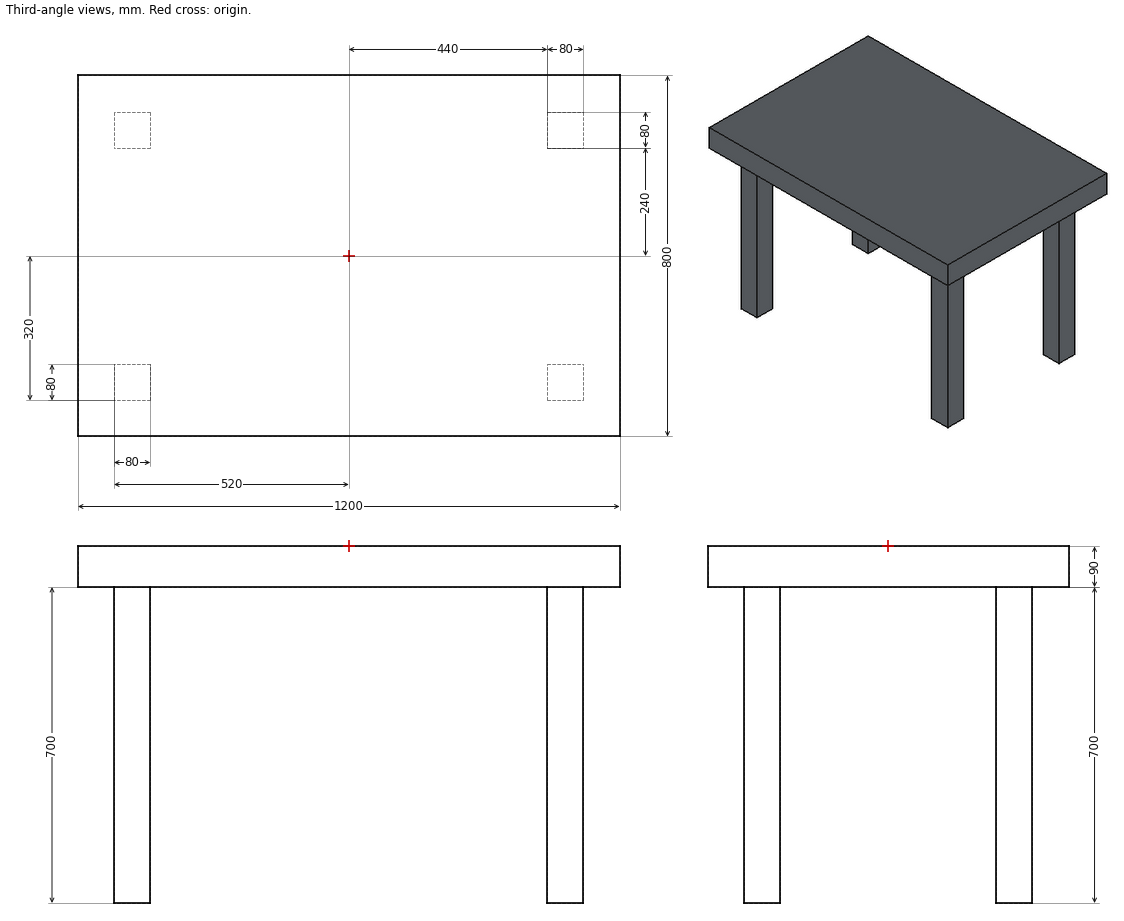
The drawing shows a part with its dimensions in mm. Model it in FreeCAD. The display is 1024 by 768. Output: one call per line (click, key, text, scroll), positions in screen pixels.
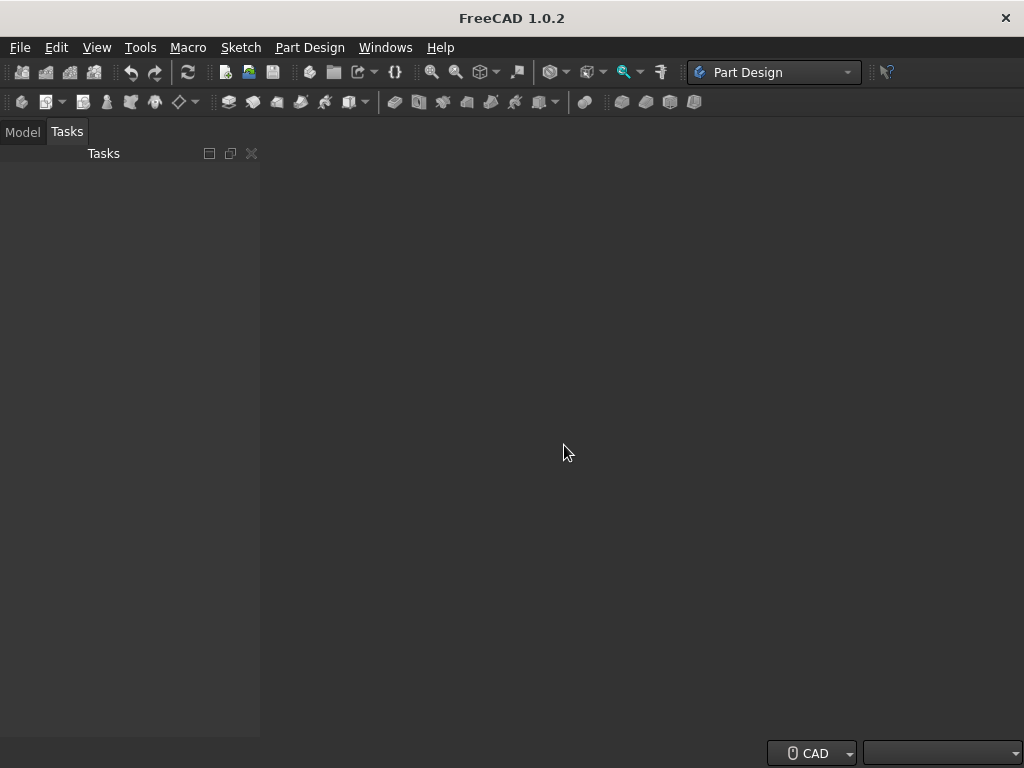
key(ctrl+n)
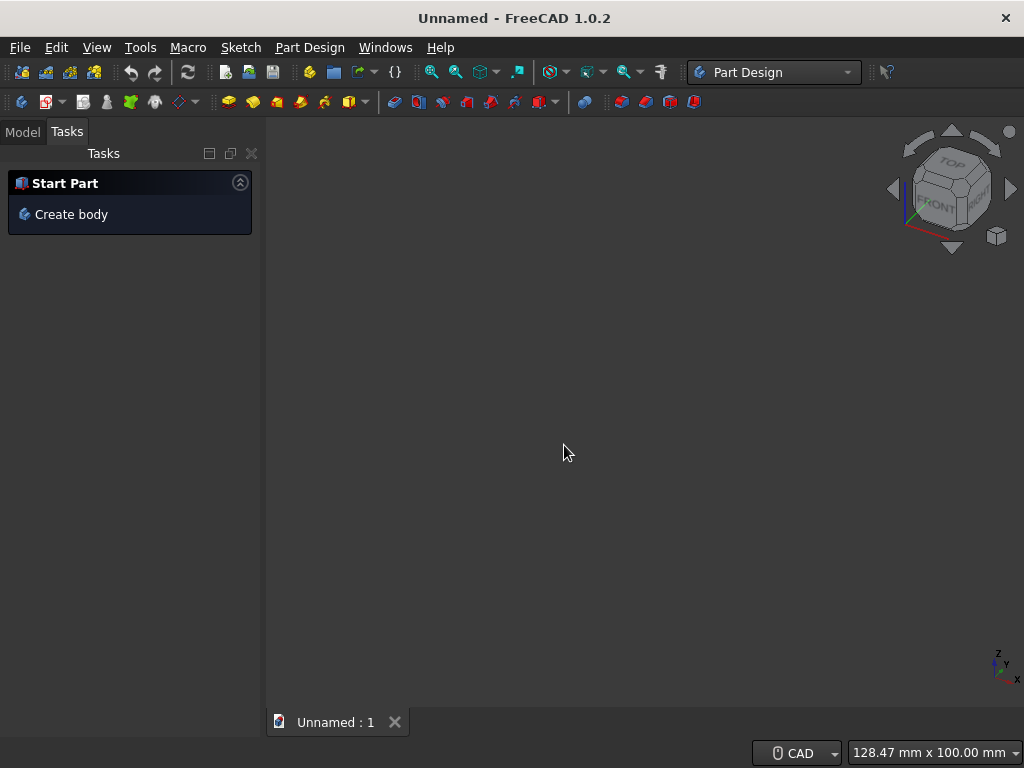
click(46, 102)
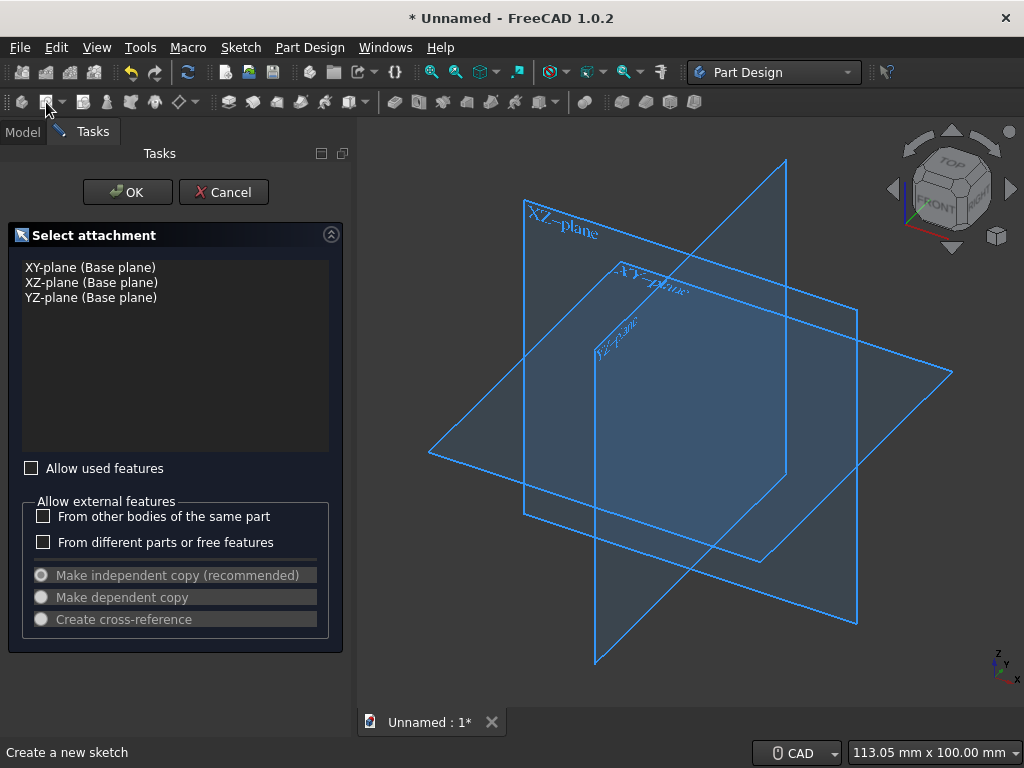
click(82, 268)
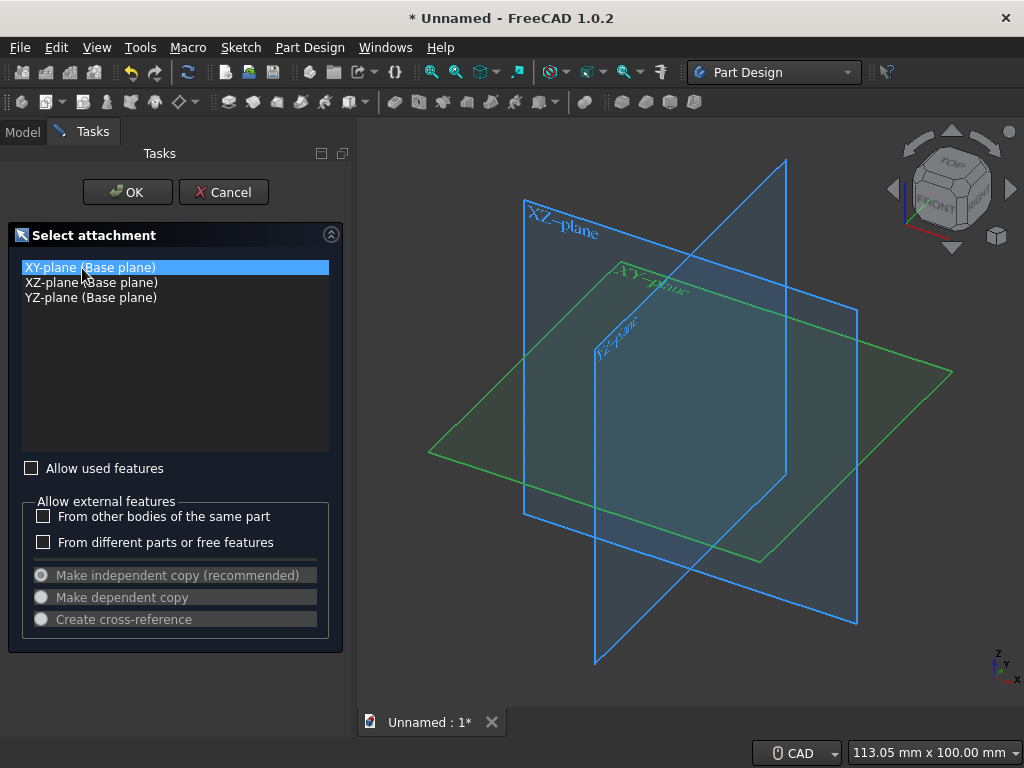
click(128, 192)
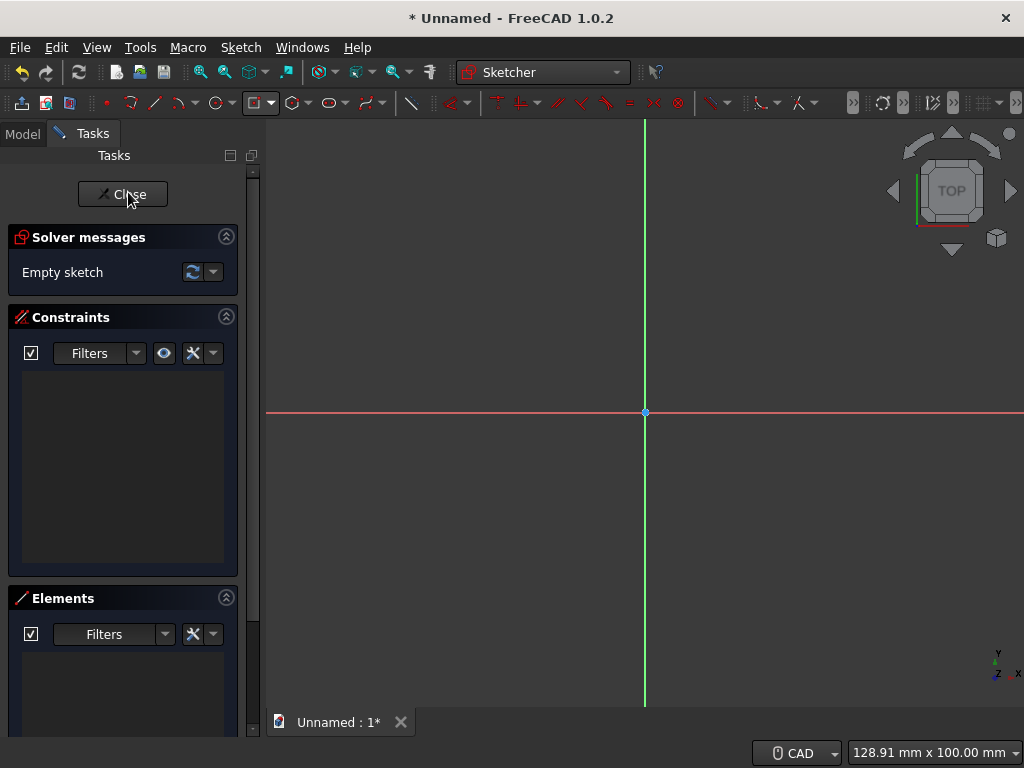
scroll(572, 413, down, 14)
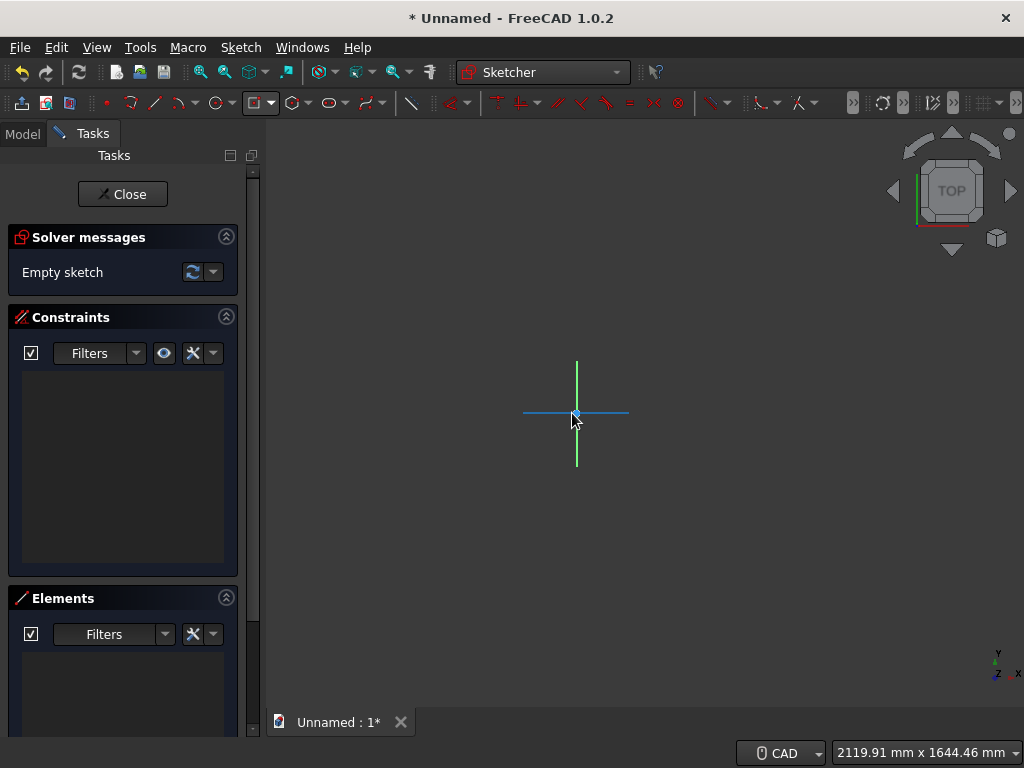
key(g)
key(v)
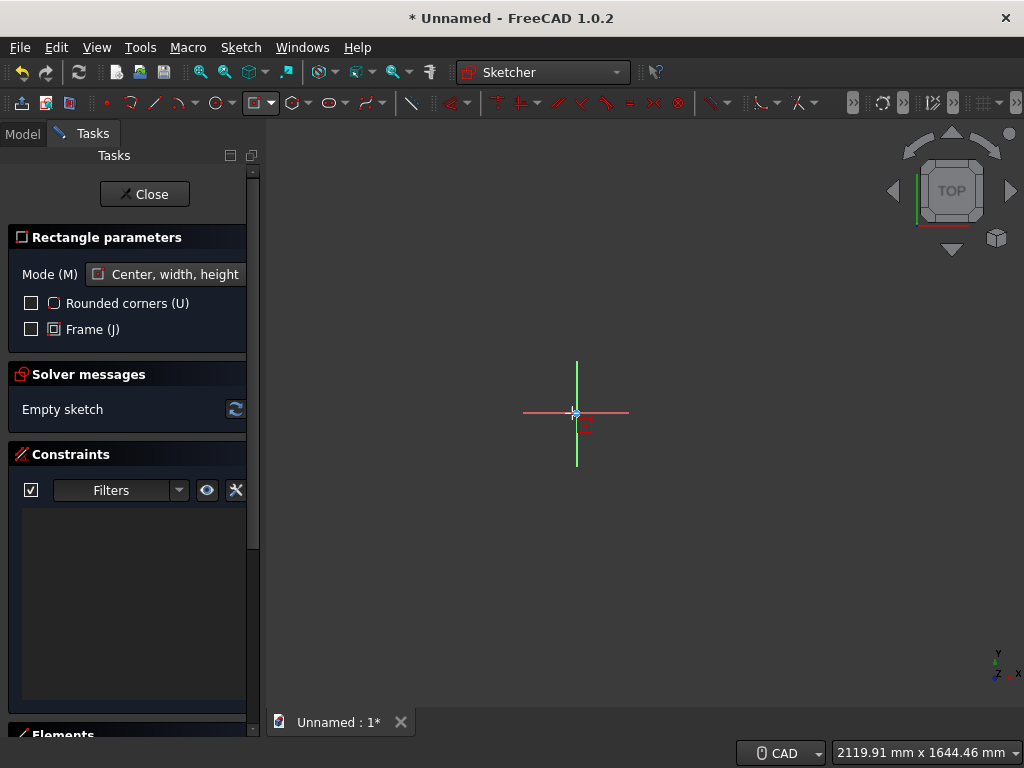
click(577, 413)
click(791, 270)
key(Escape)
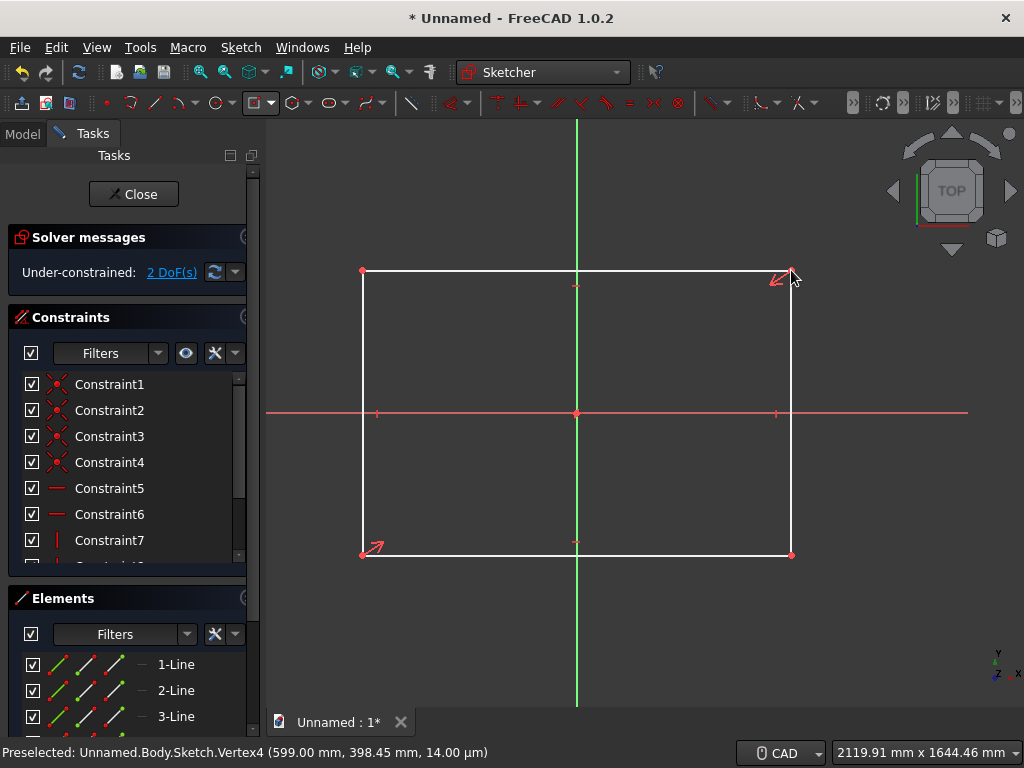
key(d)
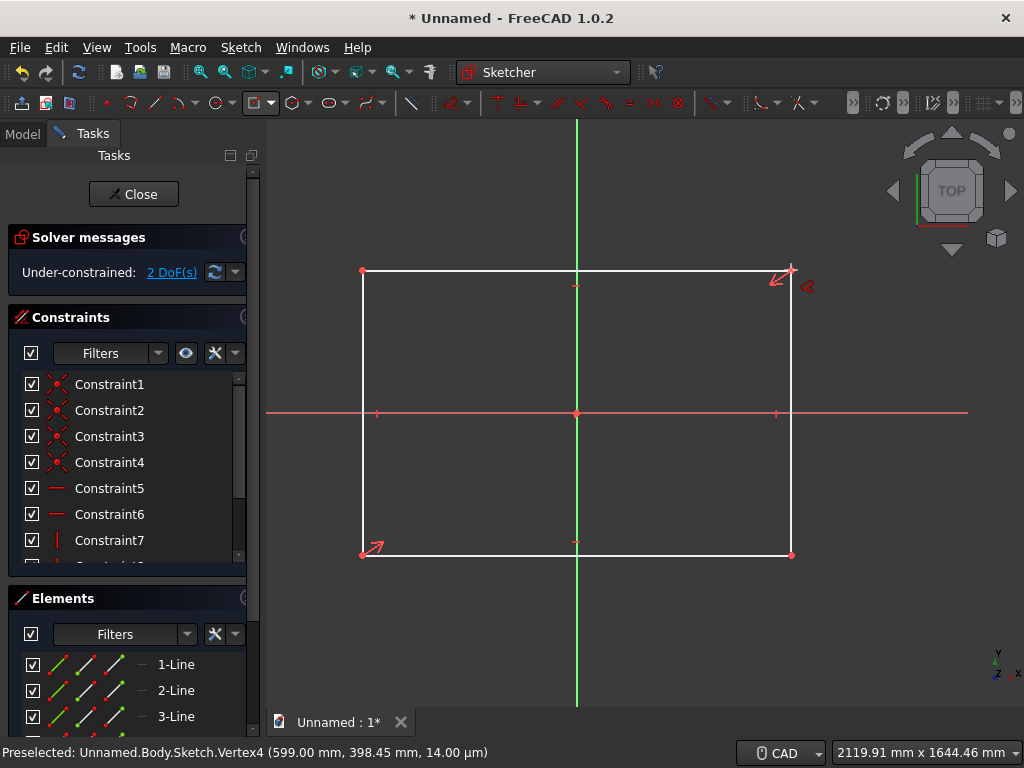
click(791, 470)
click(825, 348)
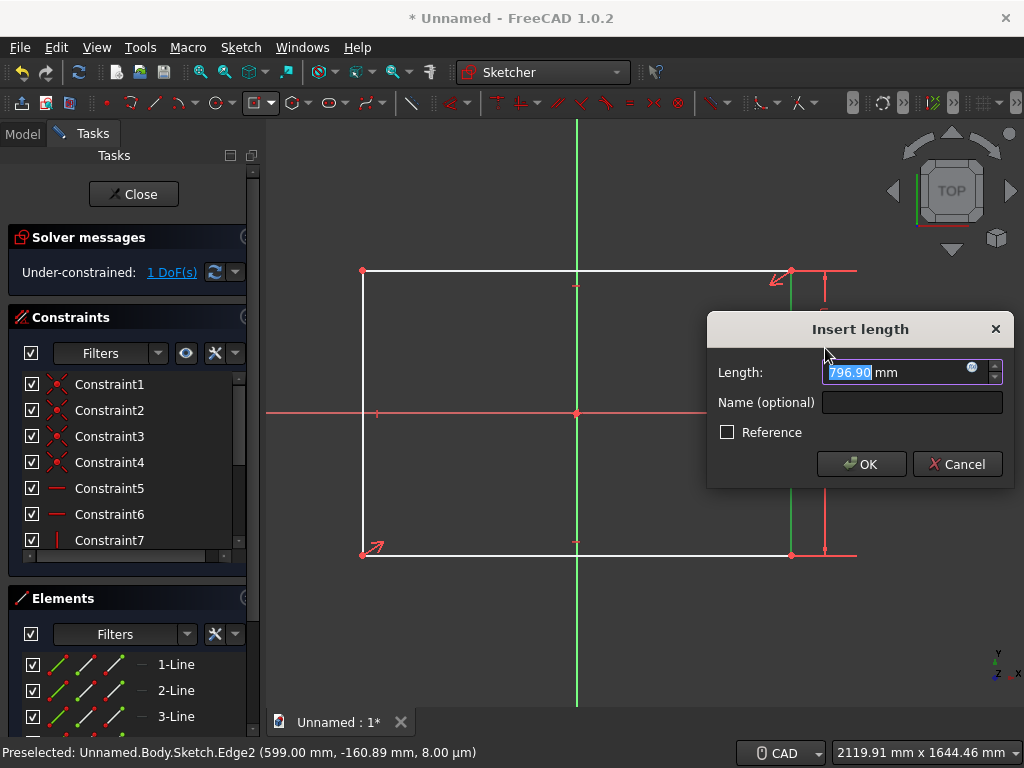
text(800)
key(Return)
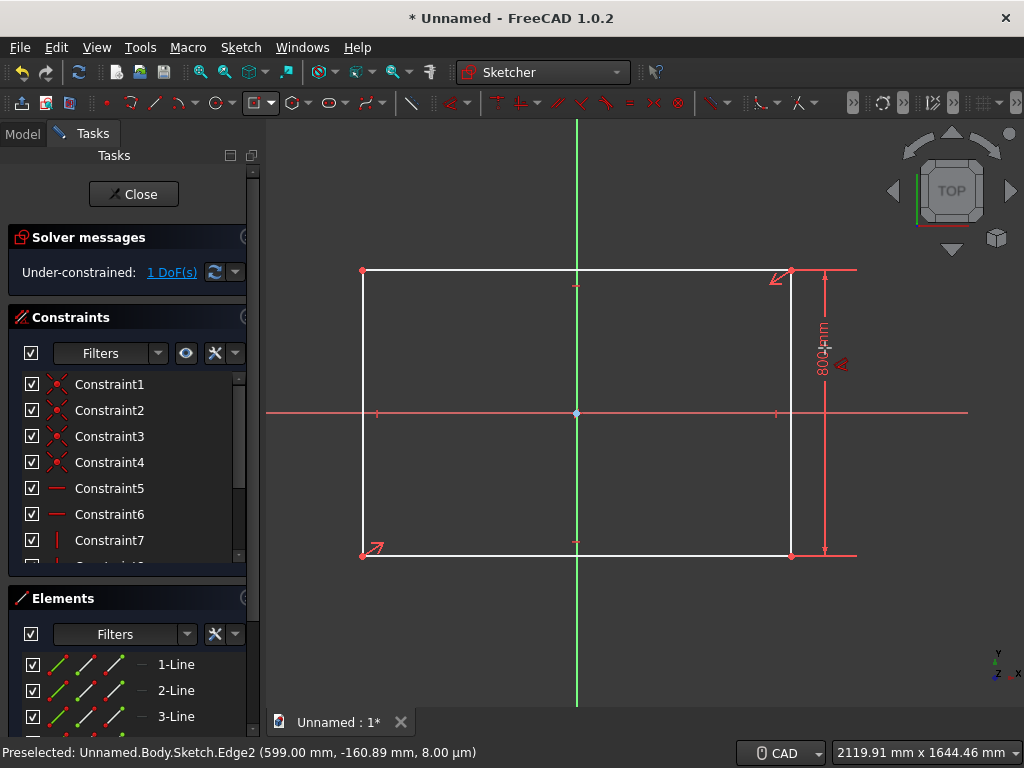
click(491, 556)
click(478, 590)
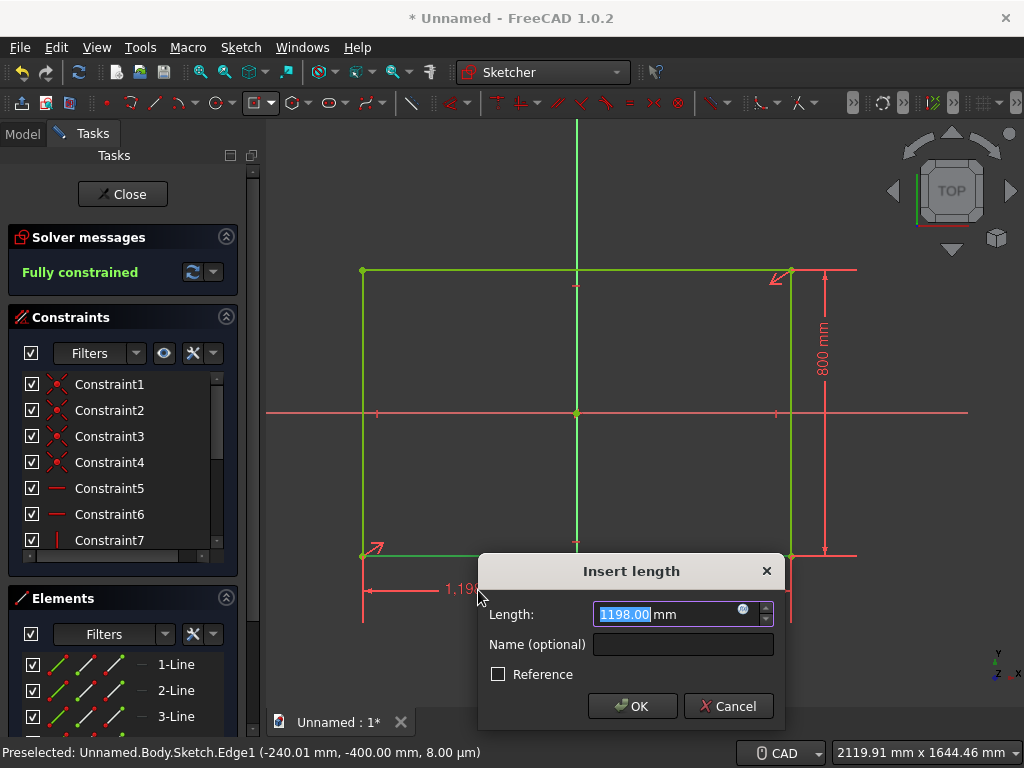
text(1200)
key(Return)
key(Escape)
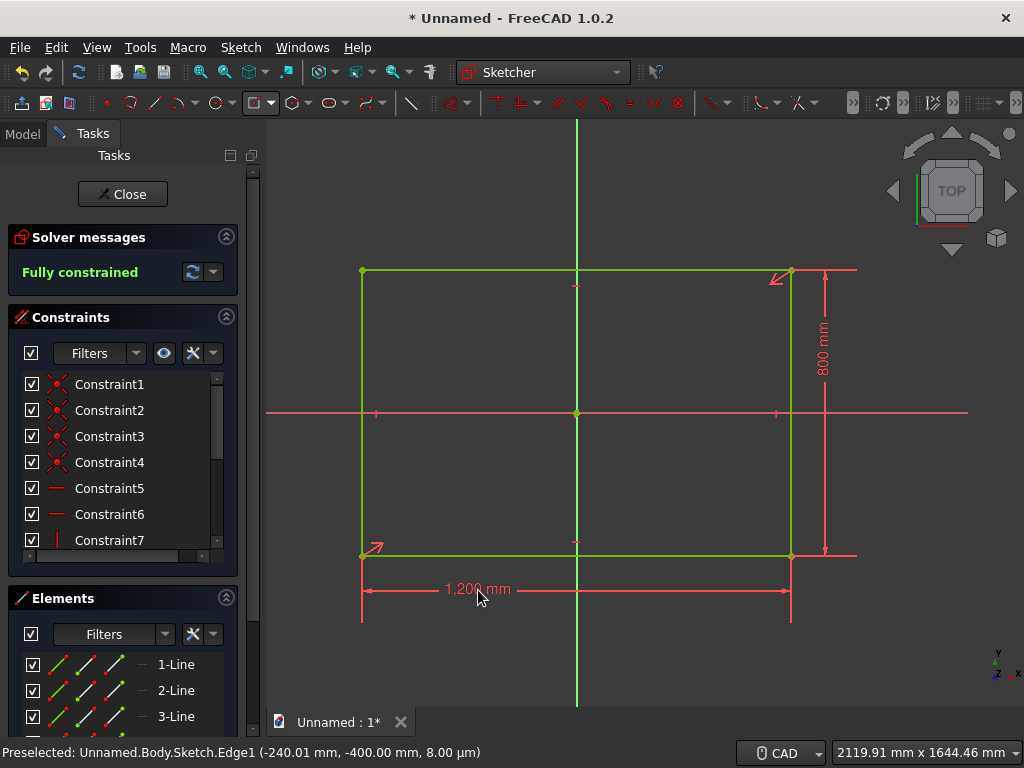
click(123, 194)